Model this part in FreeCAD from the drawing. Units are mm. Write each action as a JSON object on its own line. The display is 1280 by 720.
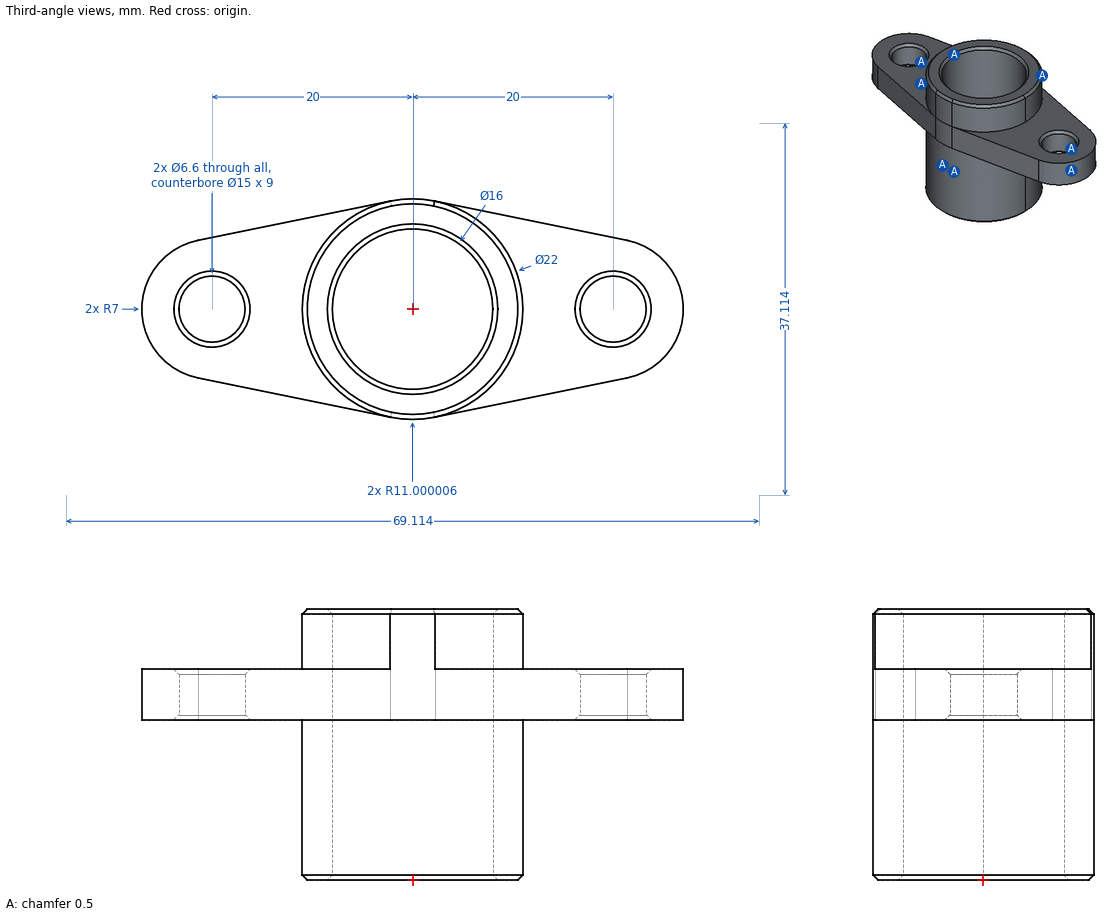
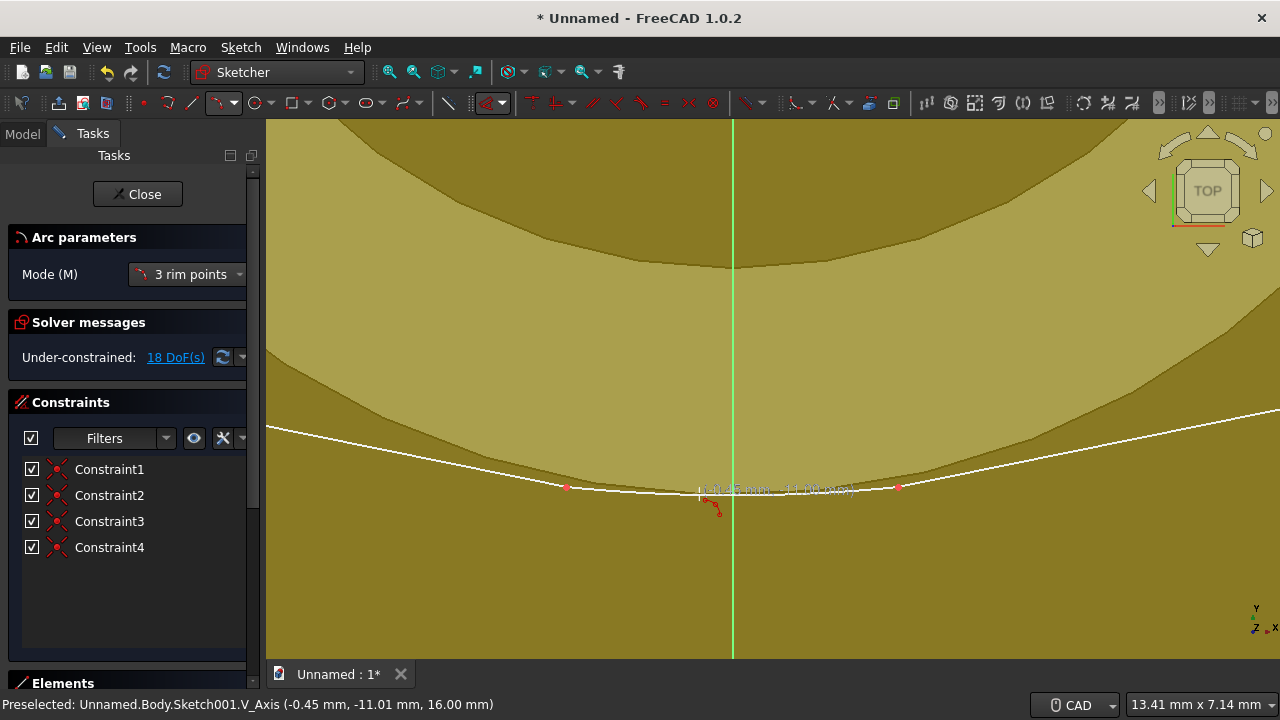
{"action": "scroll", "coordinate": [700, 503], "scroll_direction": "down", "scroll_amount": 10}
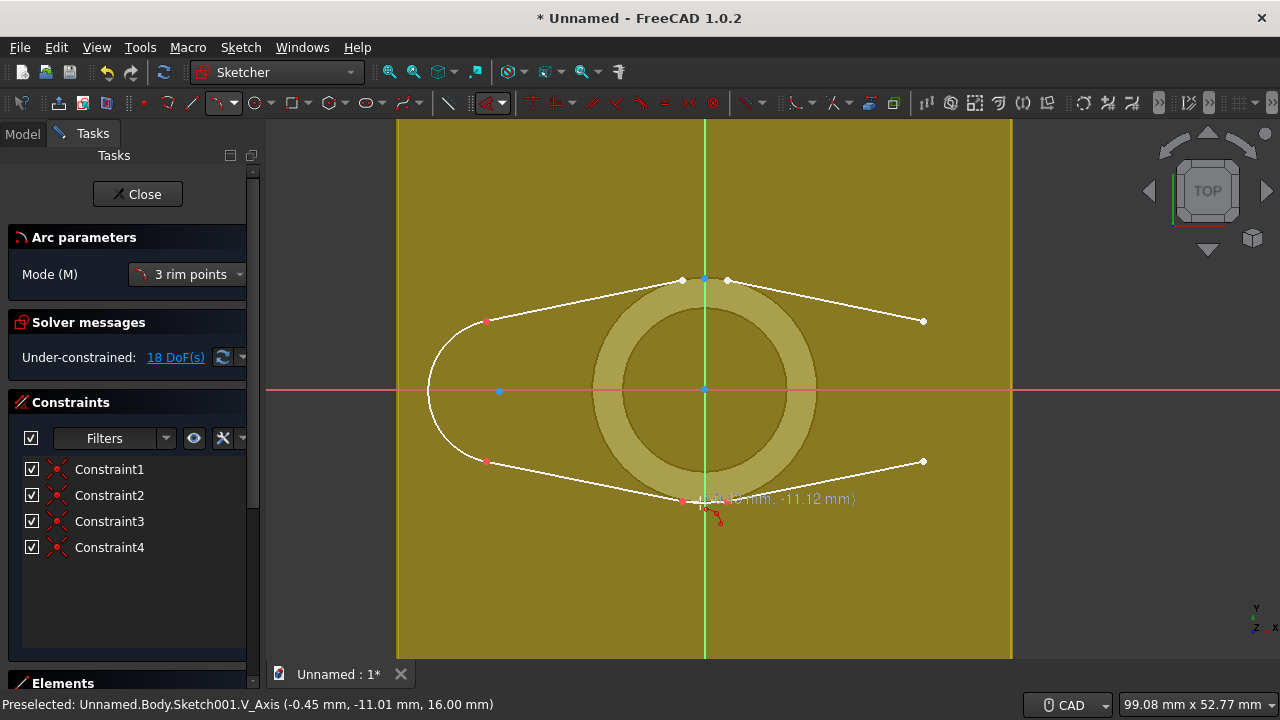
{"action": "left_click", "coordinate": [923, 462]}
{"action": "left_click", "coordinate": [923, 321]}
{"action": "left_click", "coordinate": [978, 409]}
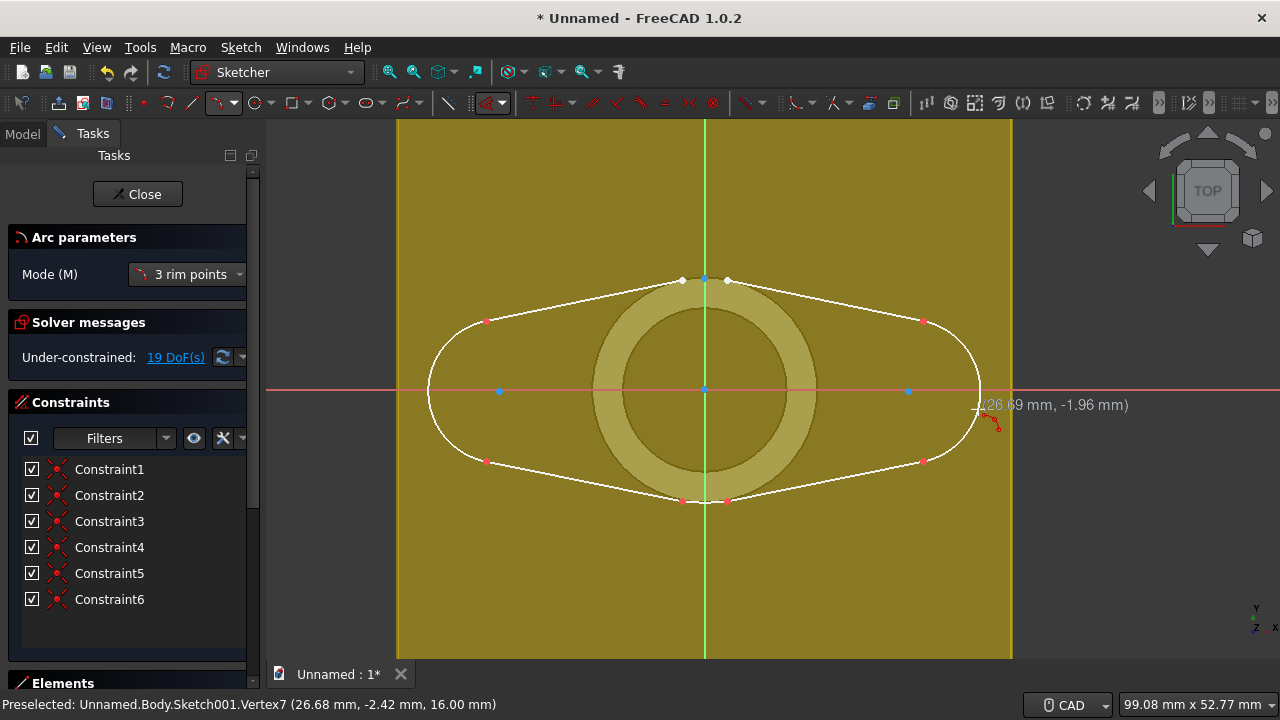
{"action": "left_click", "coordinate": [727, 280]}
{"action": "left_click", "coordinate": [682, 280]}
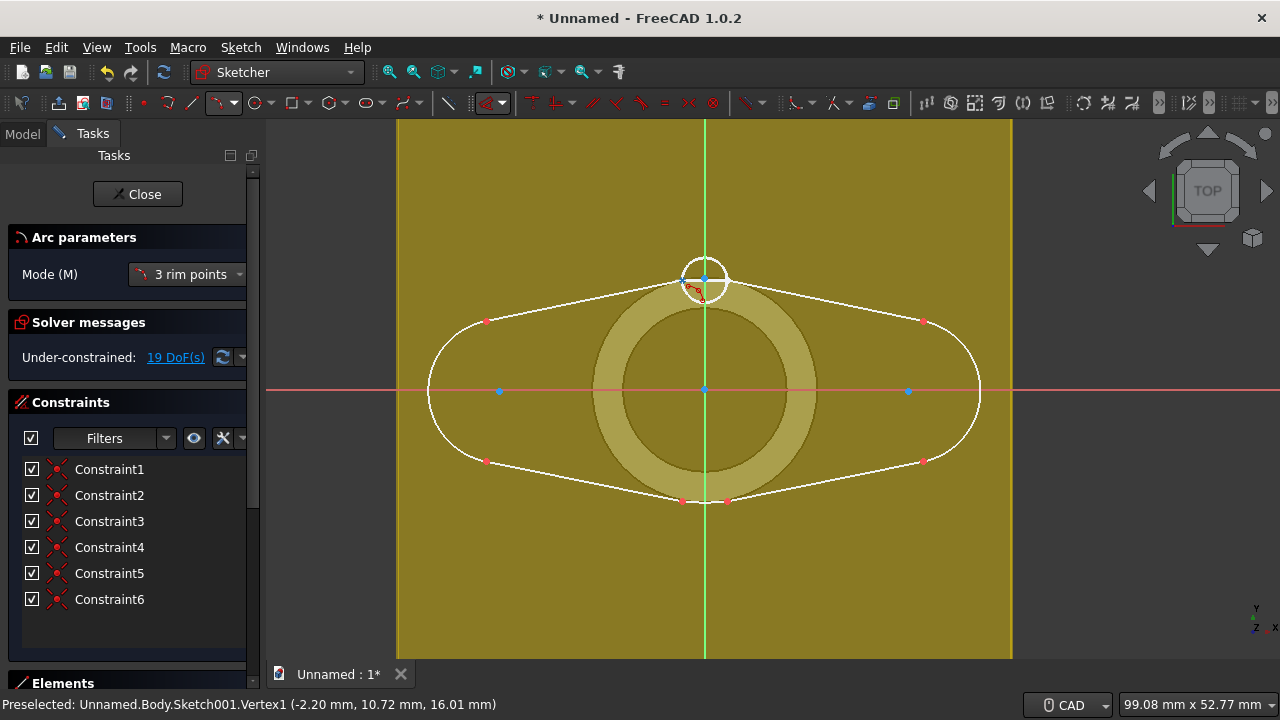
{"action": "scroll", "coordinate": [709, 277], "scroll_direction": "up", "scroll_amount": 10}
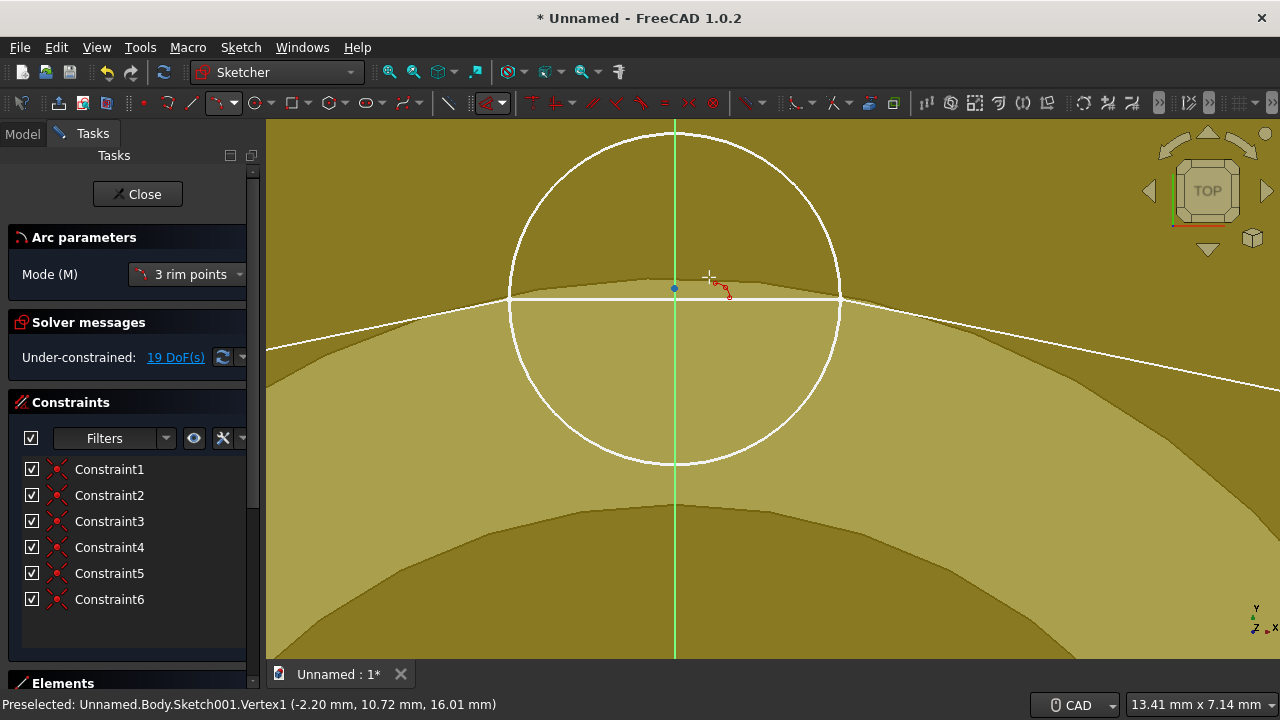
{"action": "left_click", "coordinate": [709, 279]}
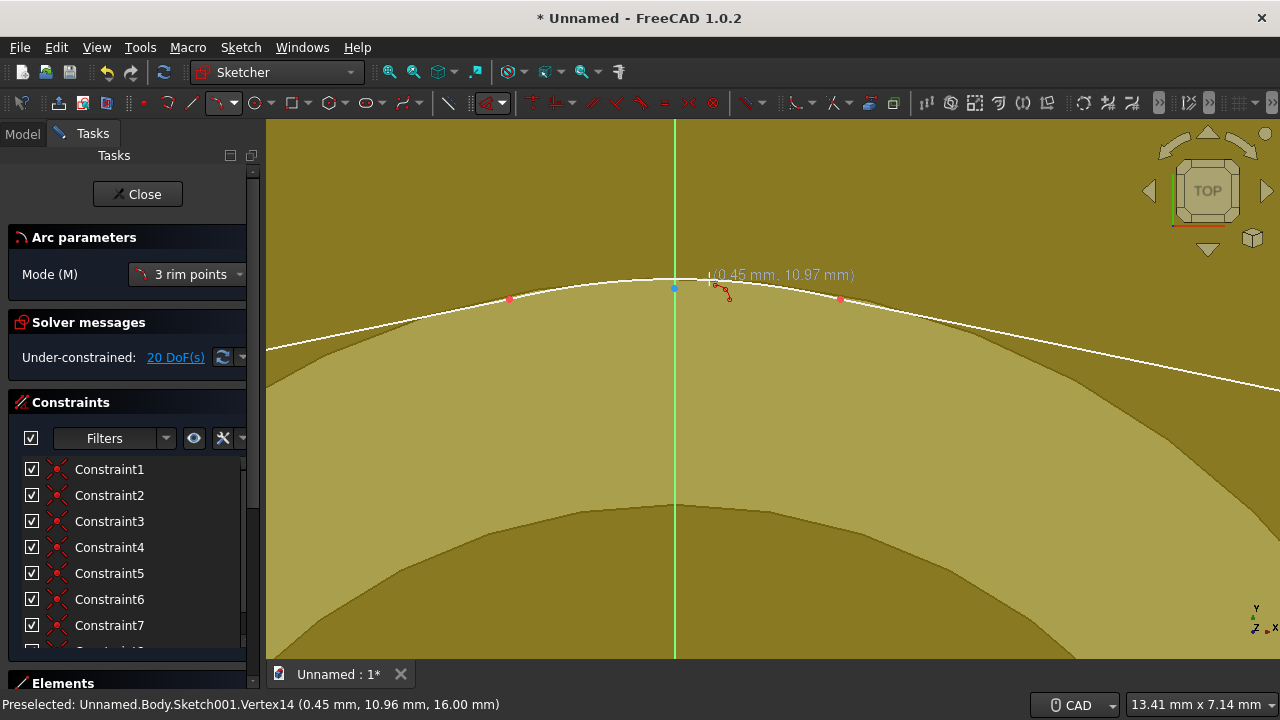
{"action": "left_click", "coordinate": [256, 104]}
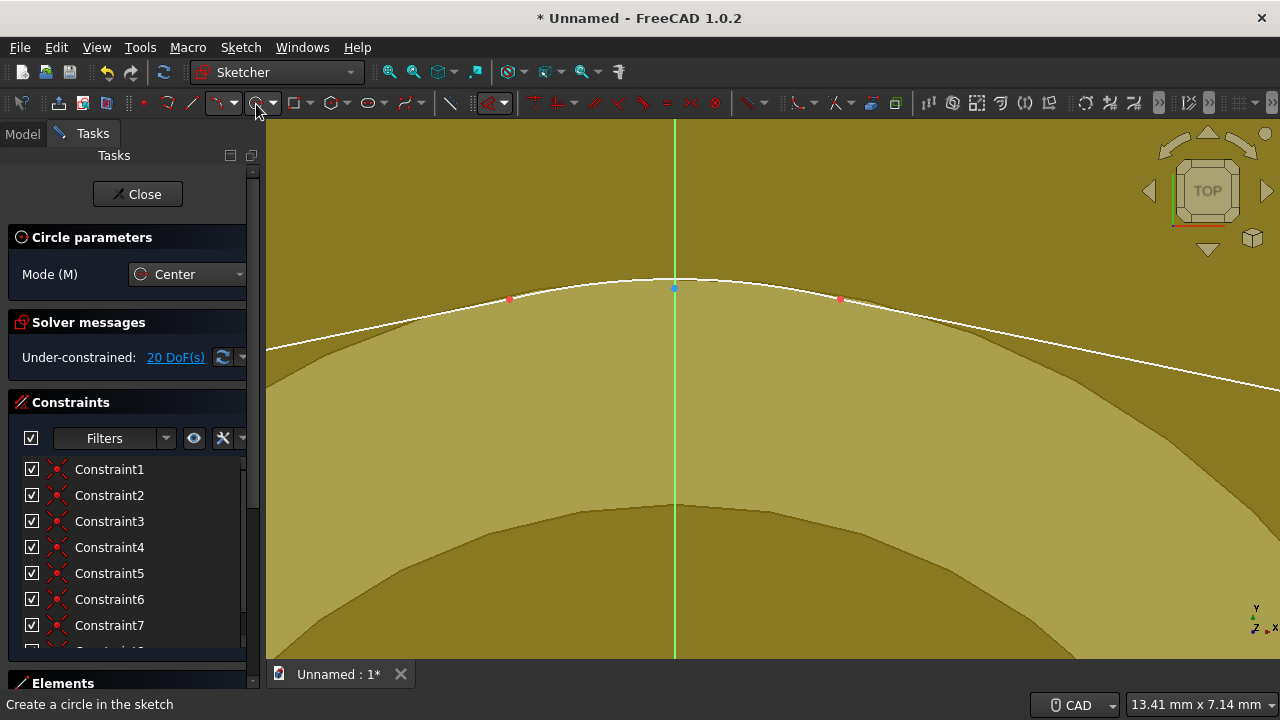
{"action": "scroll", "coordinate": [709, 276], "scroll_direction": "down", "scroll_amount": 10}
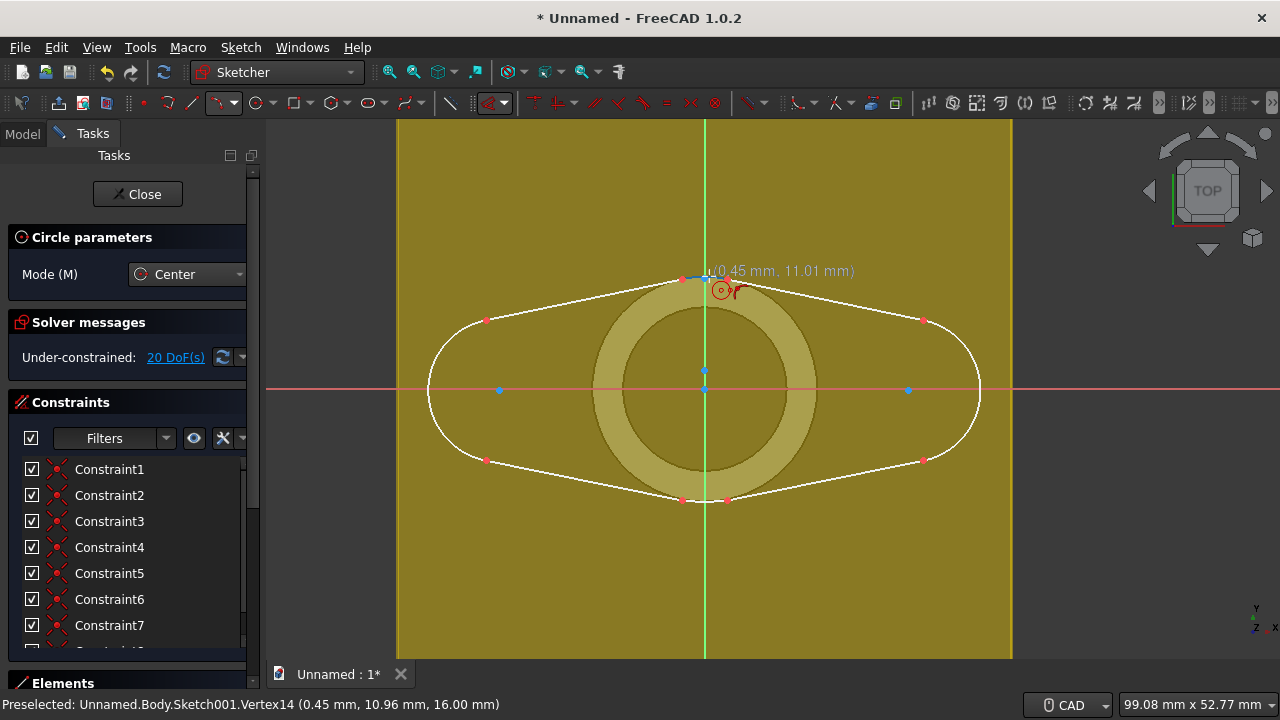
{"action": "left_click", "coordinate": [705, 389]}
{"action": "left_click", "coordinate": [763, 331]}
{"action": "key", "text": "Escape"}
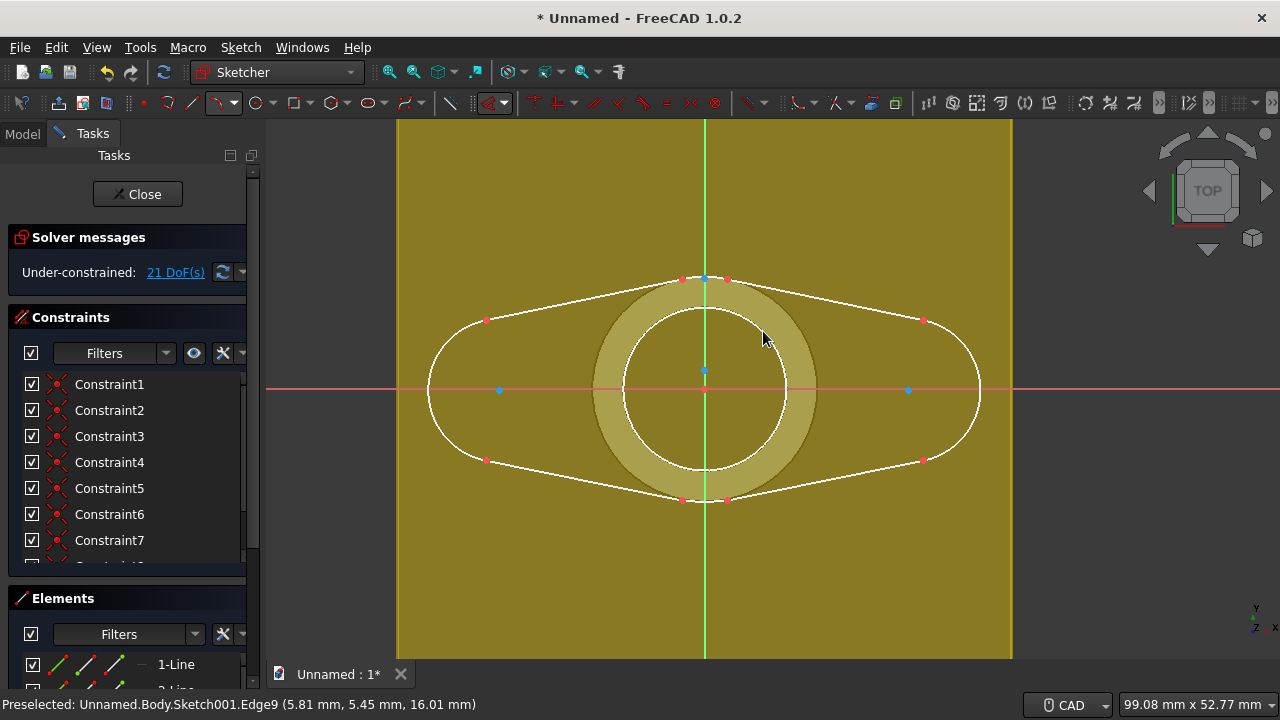
{"action": "left_click", "coordinate": [623, 292]}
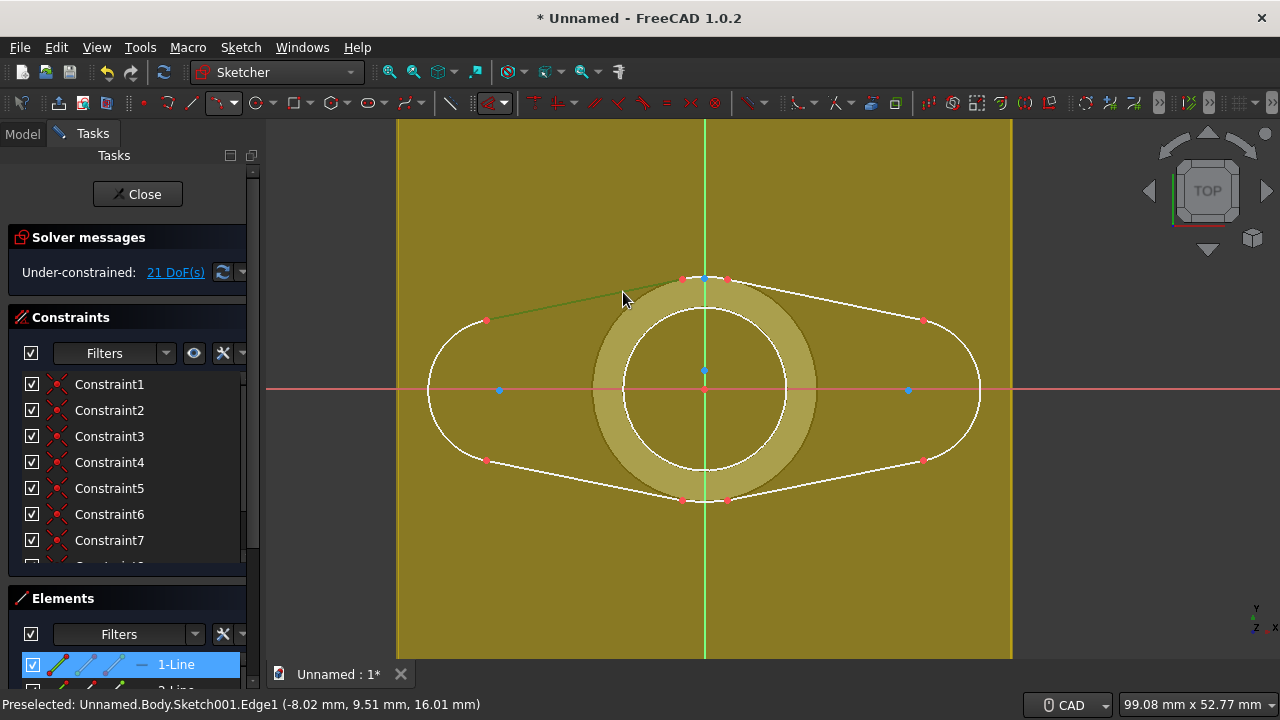
{"action": "left_click", "coordinate": [439, 353]}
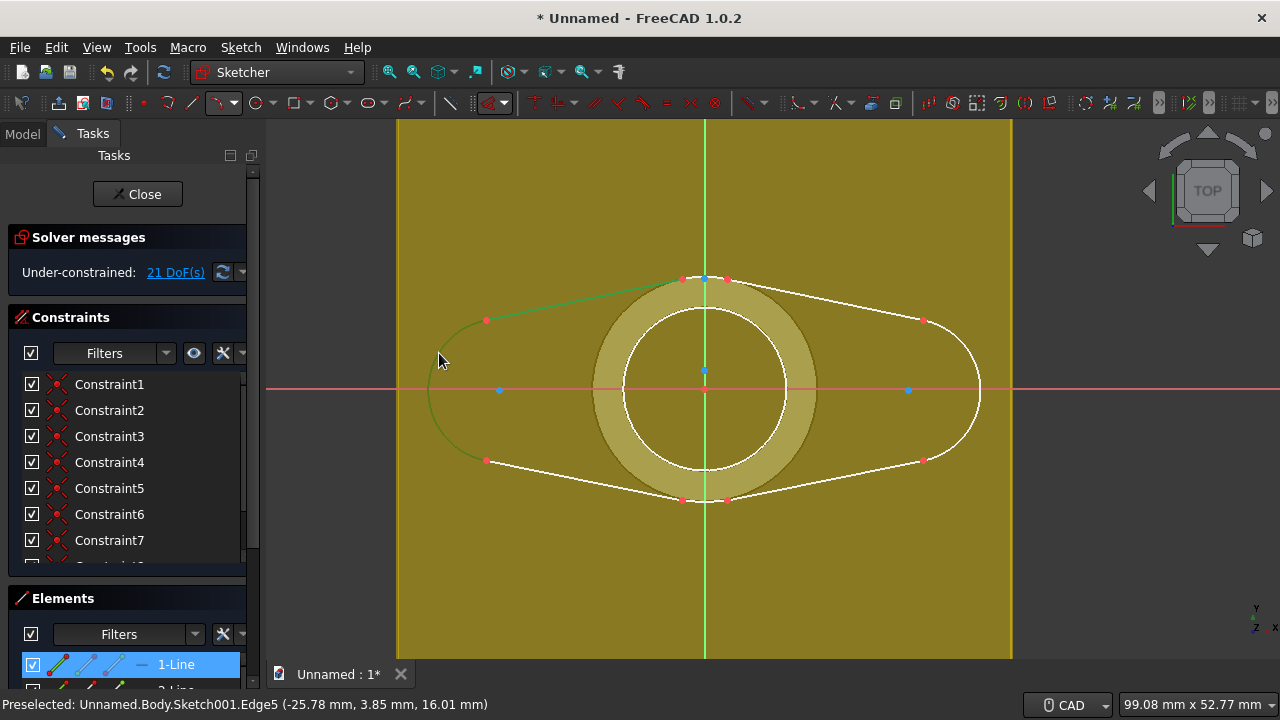
{"action": "key", "text": "t"}